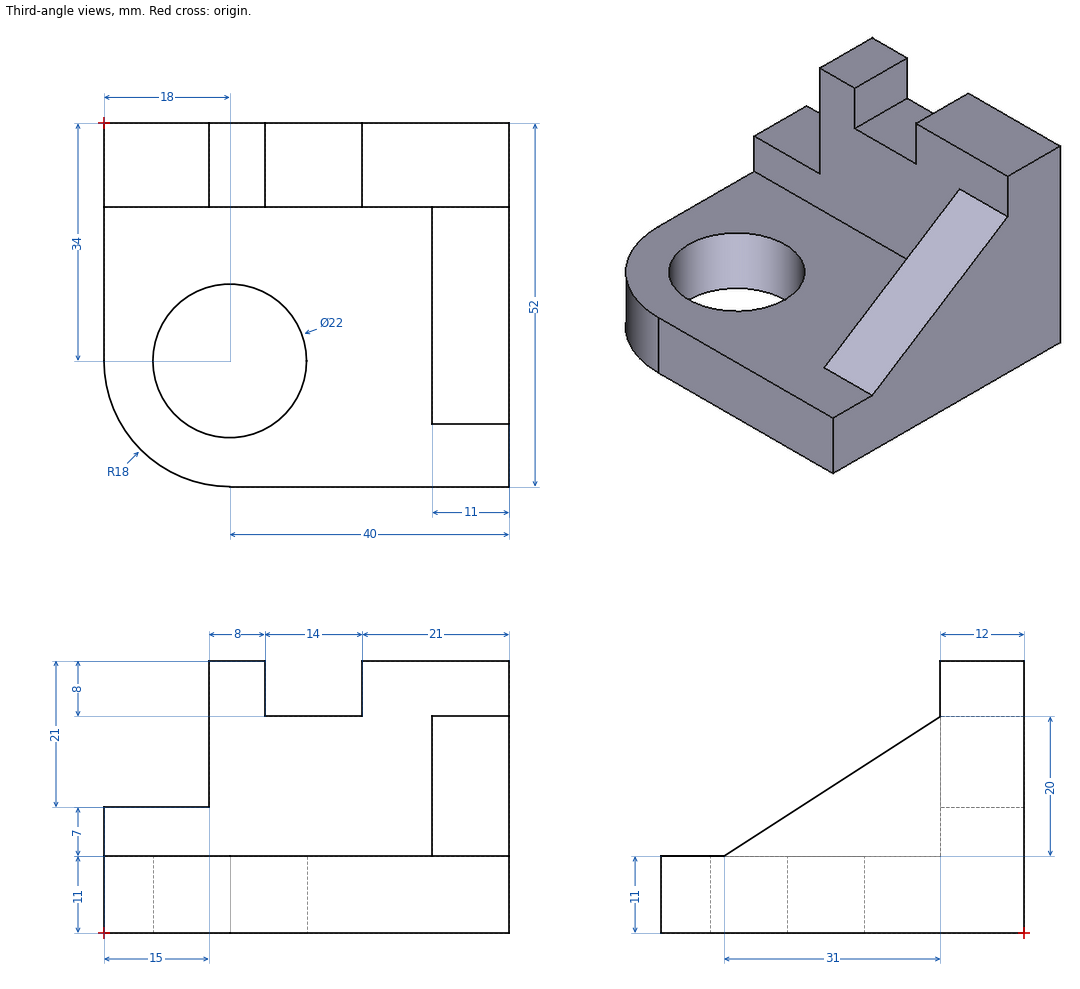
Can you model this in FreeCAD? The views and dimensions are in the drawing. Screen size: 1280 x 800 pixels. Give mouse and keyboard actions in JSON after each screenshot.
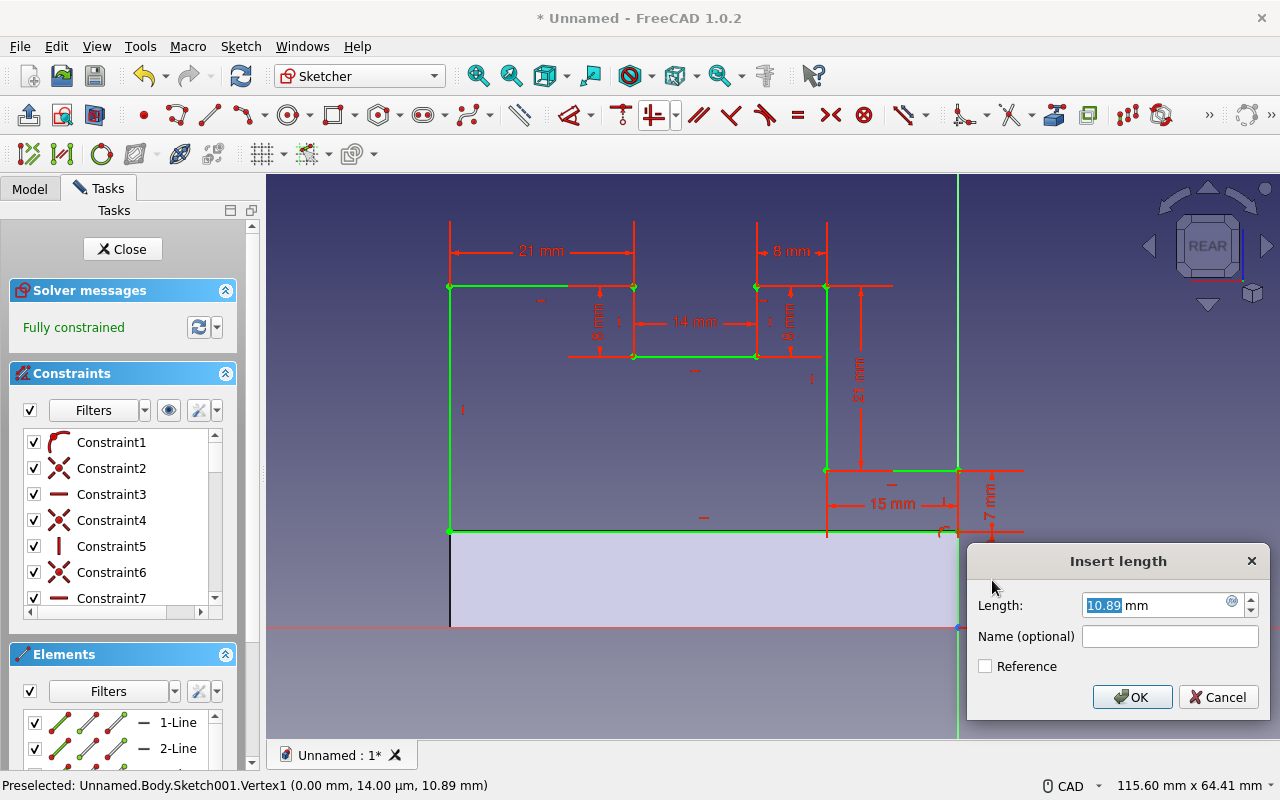
{"action": "type", "text": "11"}
{"action": "key", "text": "Return"}
{"action": "key", "text": "Escape"}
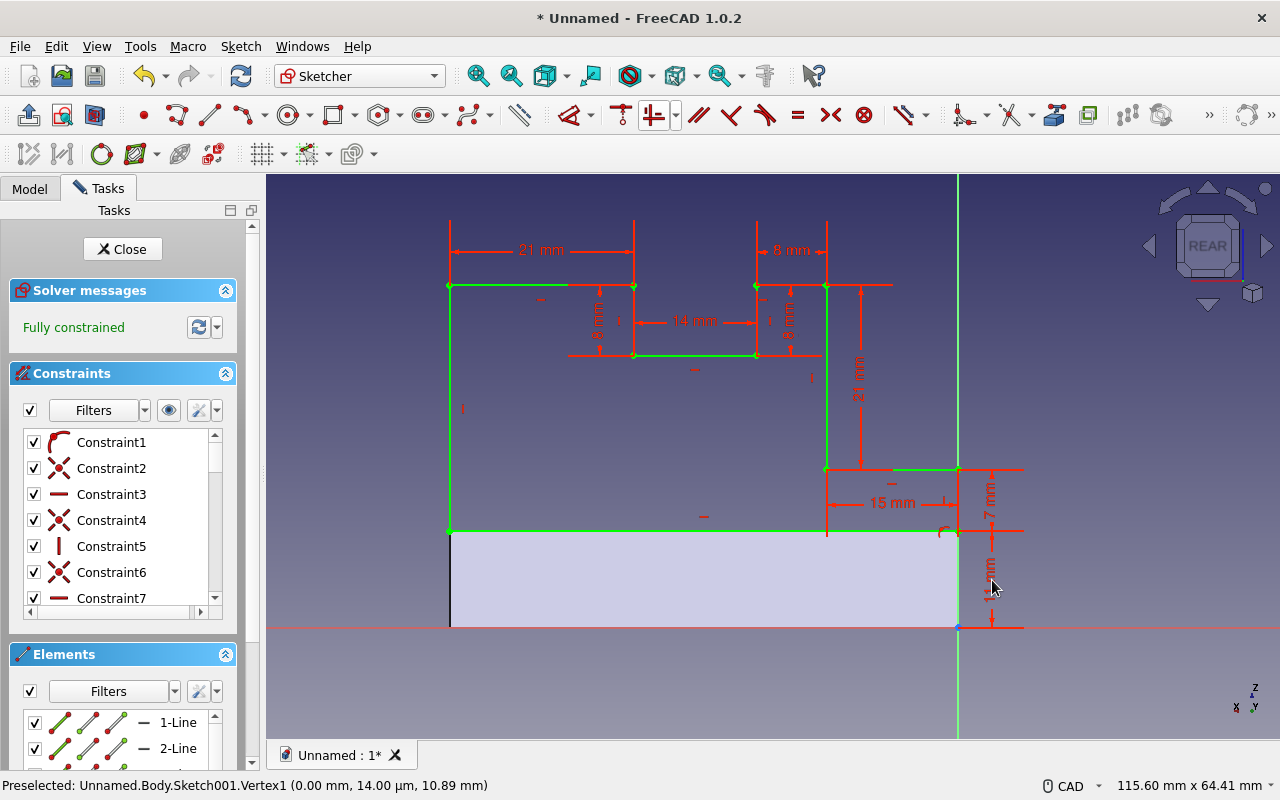
{"action": "left_click", "coordinate": [123, 249]}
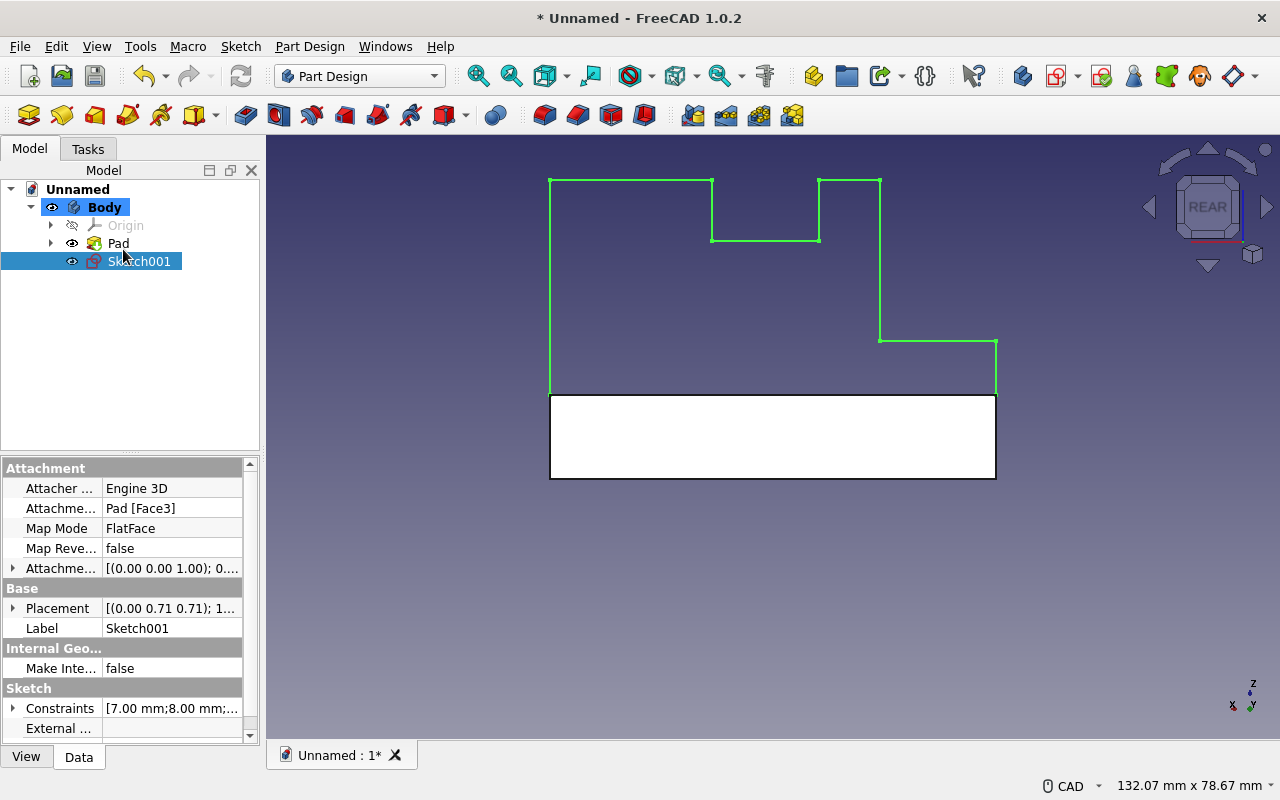
{"action": "left_click", "coordinate": [29, 116]}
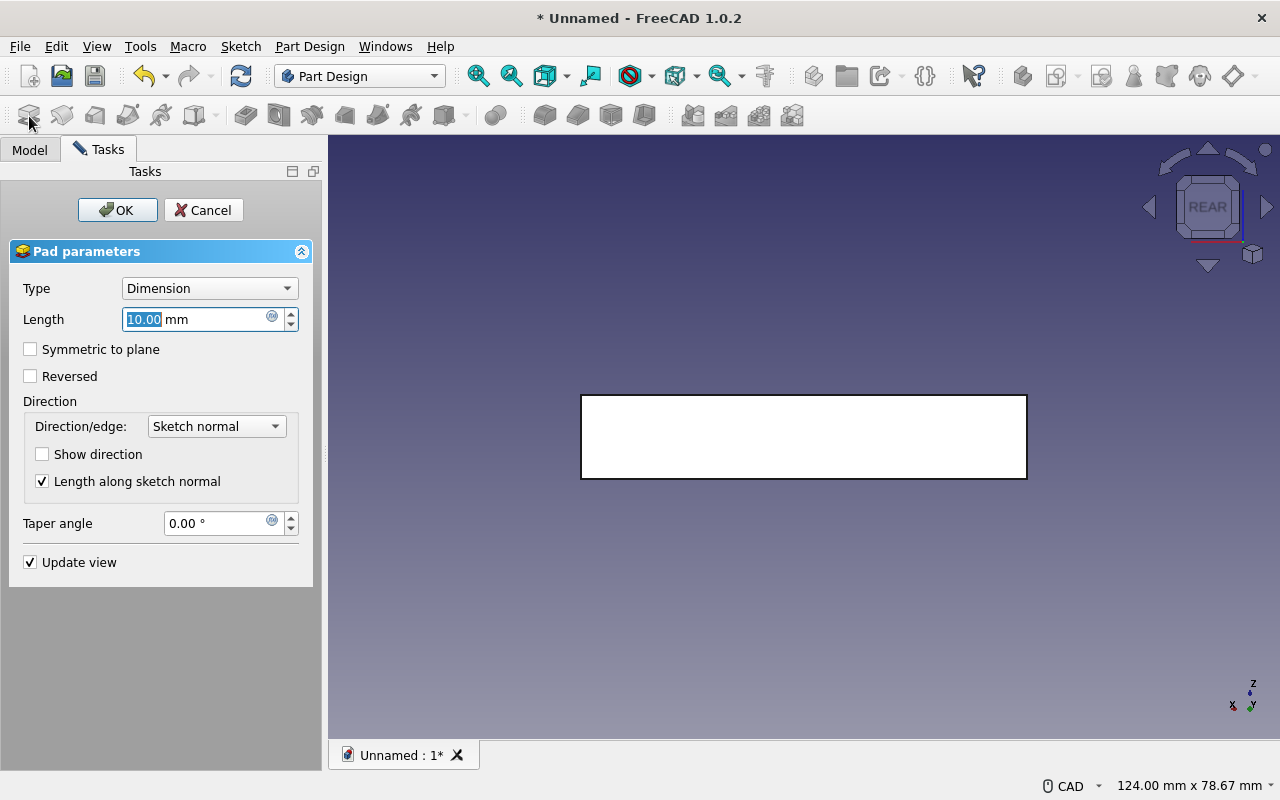
{"action": "type", "text": "12"}
{"action": "key", "text": "Tab"}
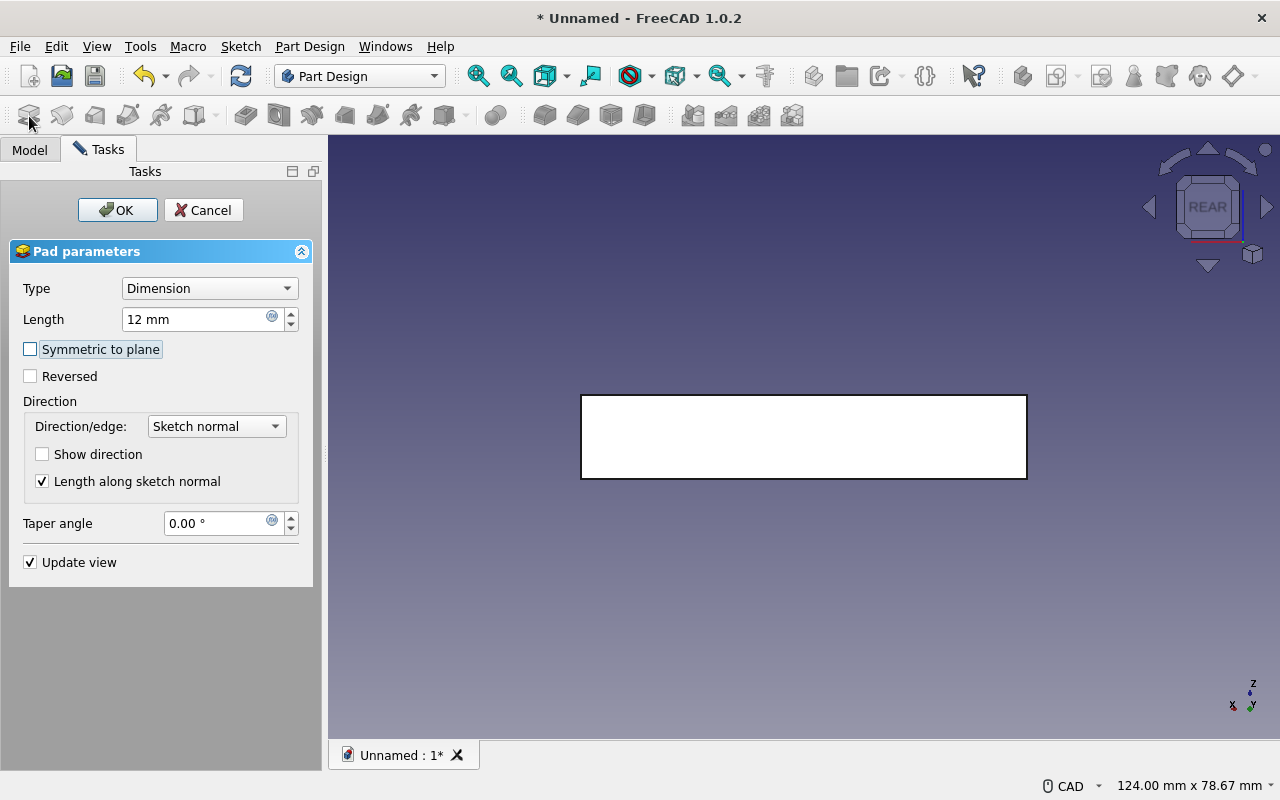
{"action": "left_click", "coordinate": [31, 376]}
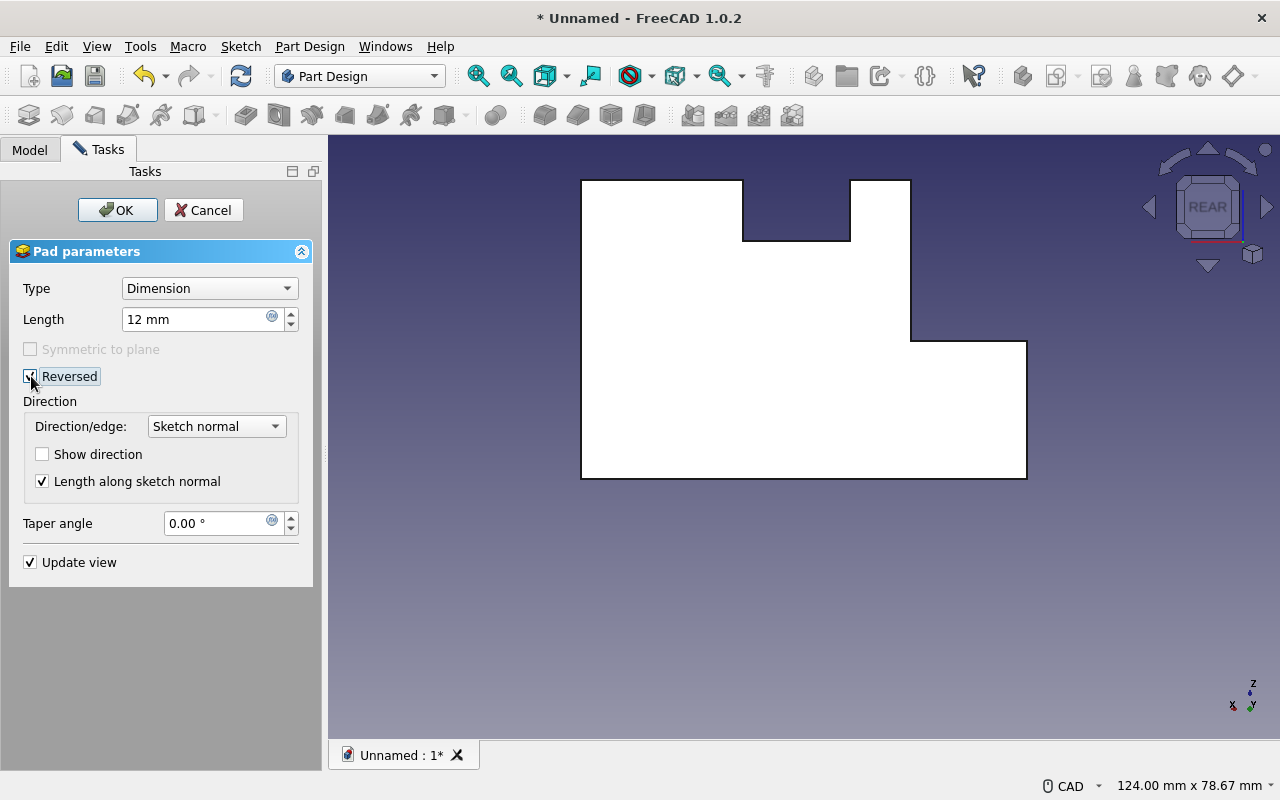
{"action": "left_click", "coordinate": [118, 210]}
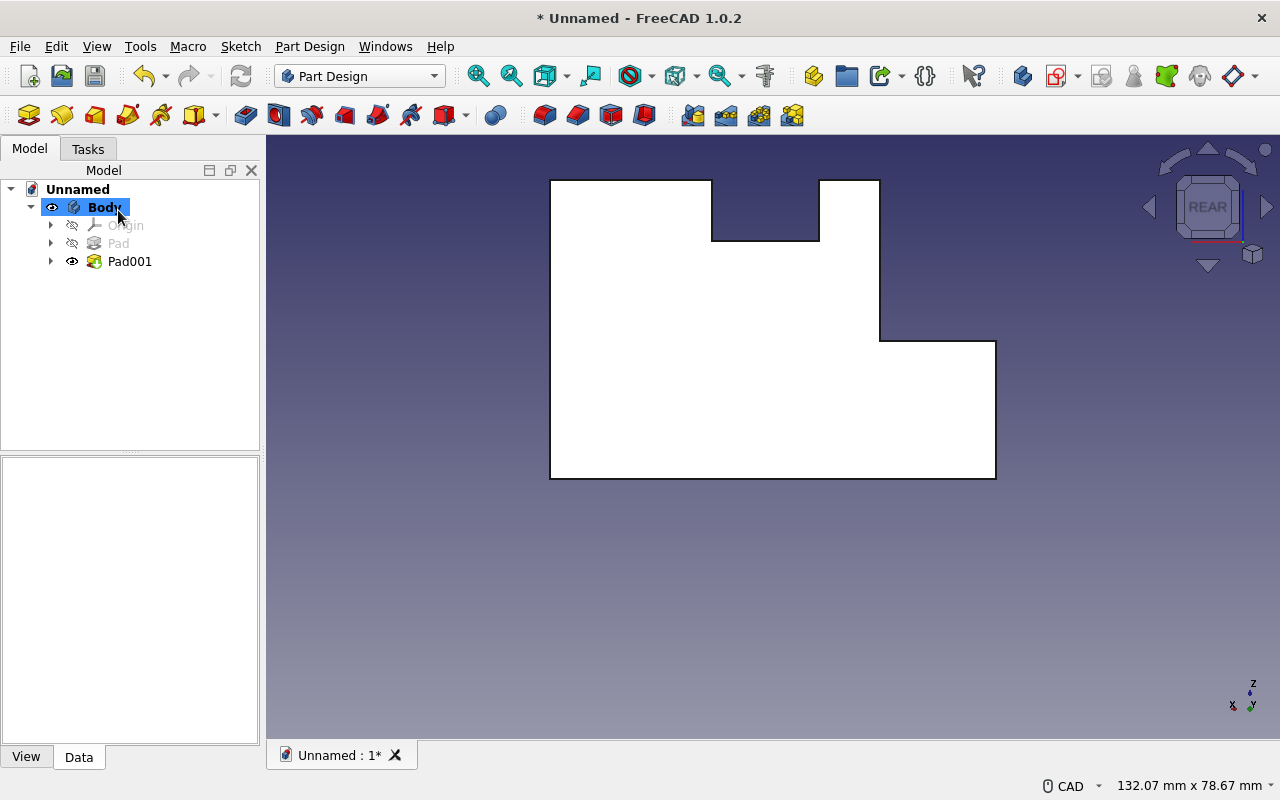
{"action": "key", "text": "0"}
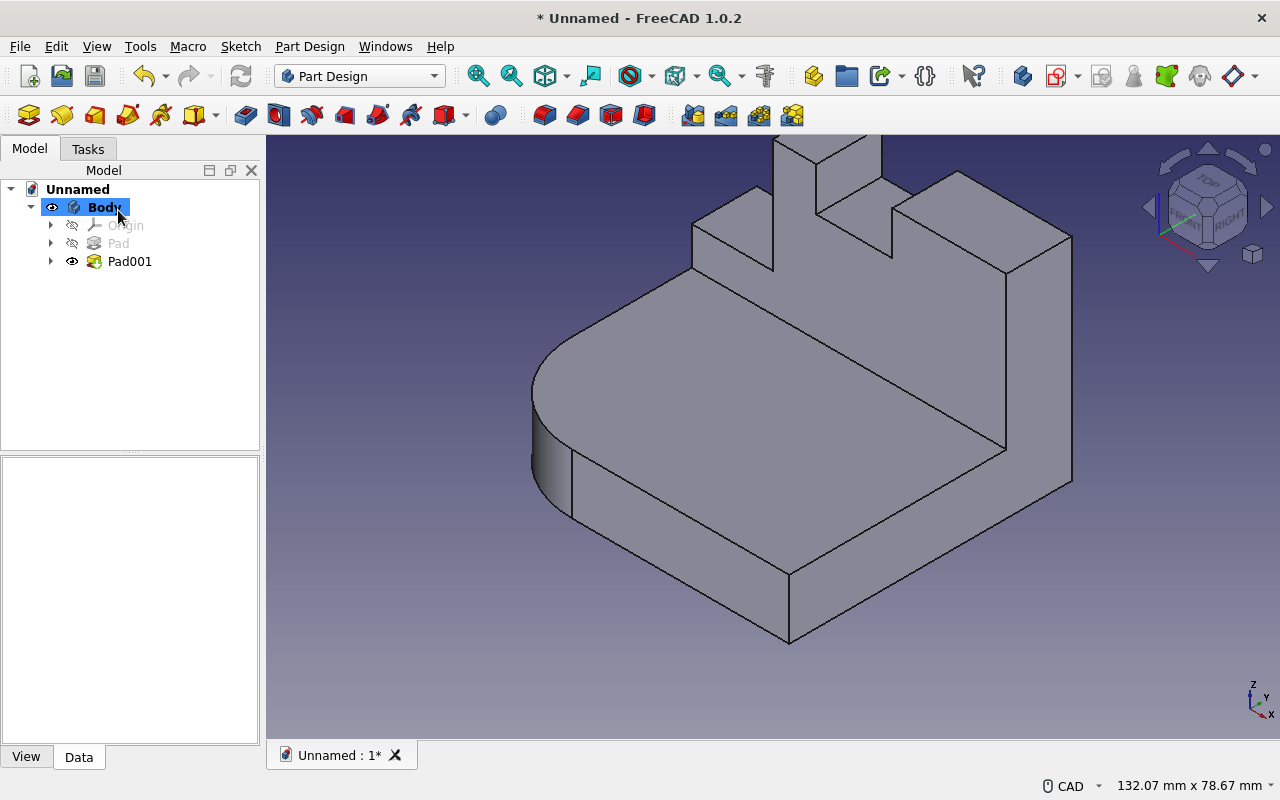
{"action": "left_click", "coordinate": [479, 76]}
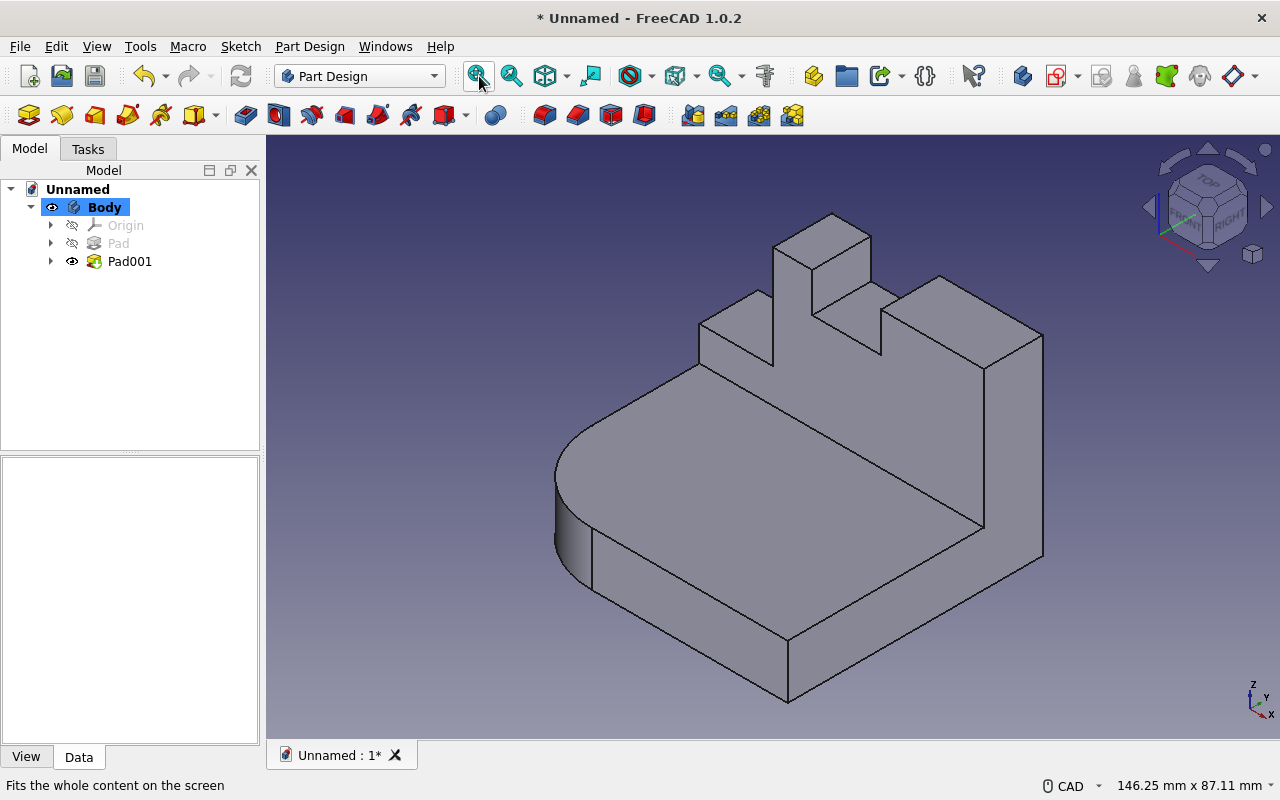
{"action": "left_click", "coordinate": [1024, 392]}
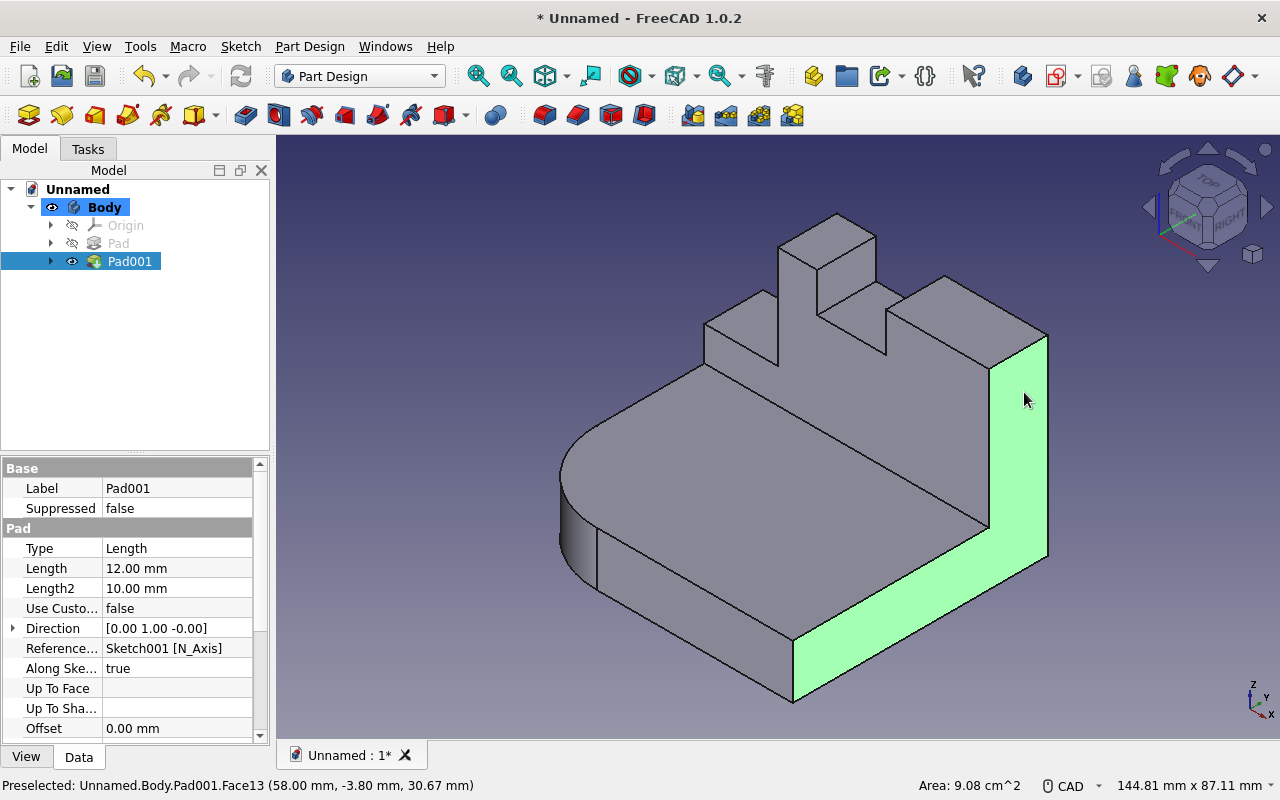
{"action": "left_click", "coordinate": [1056, 76]}